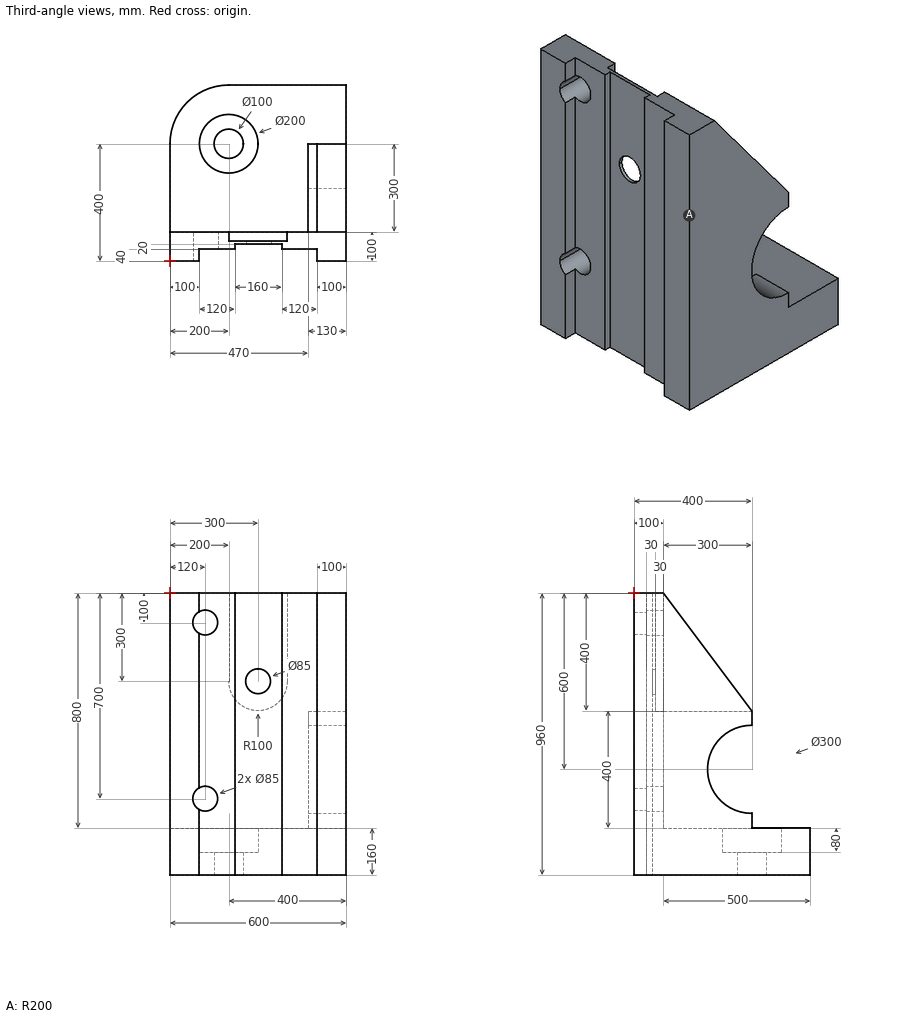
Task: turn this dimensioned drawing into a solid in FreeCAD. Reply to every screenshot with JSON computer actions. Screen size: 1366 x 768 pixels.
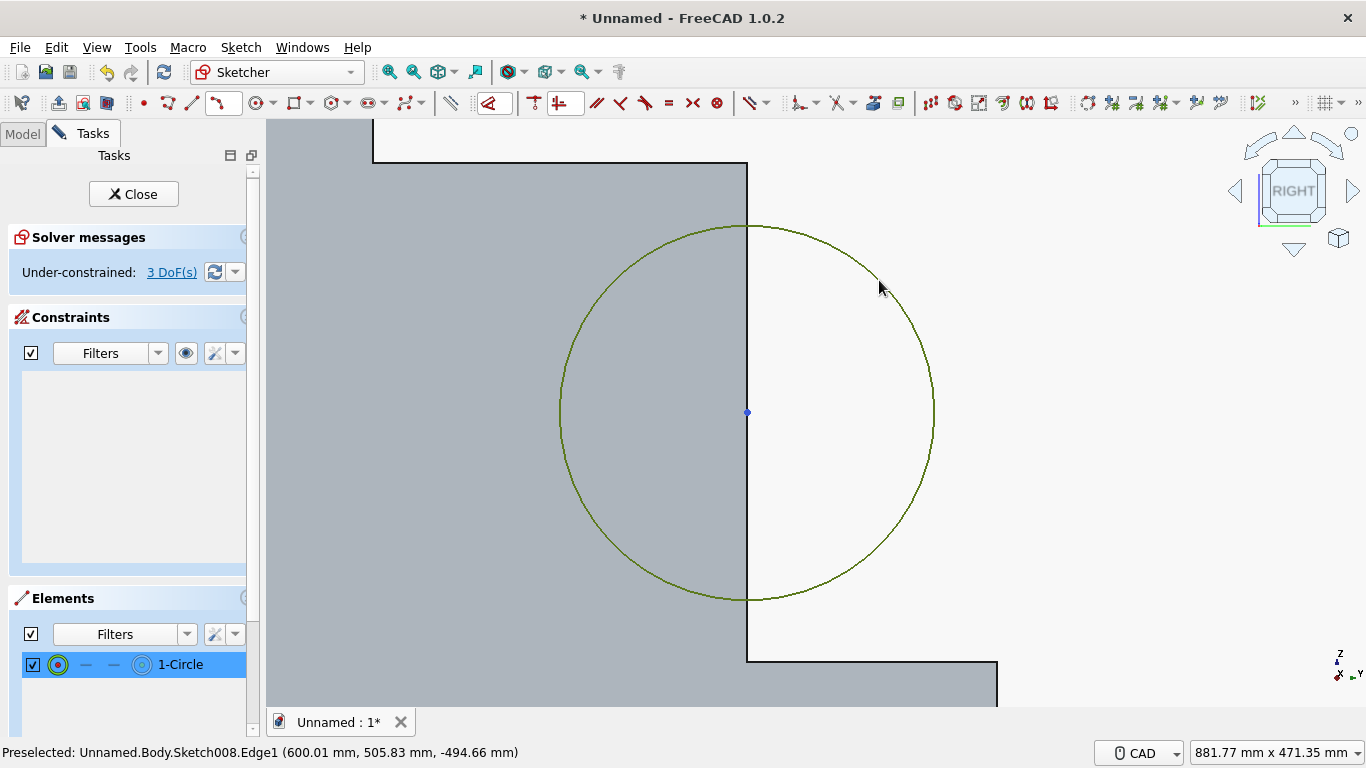
{"action": "key", "text": "k o"}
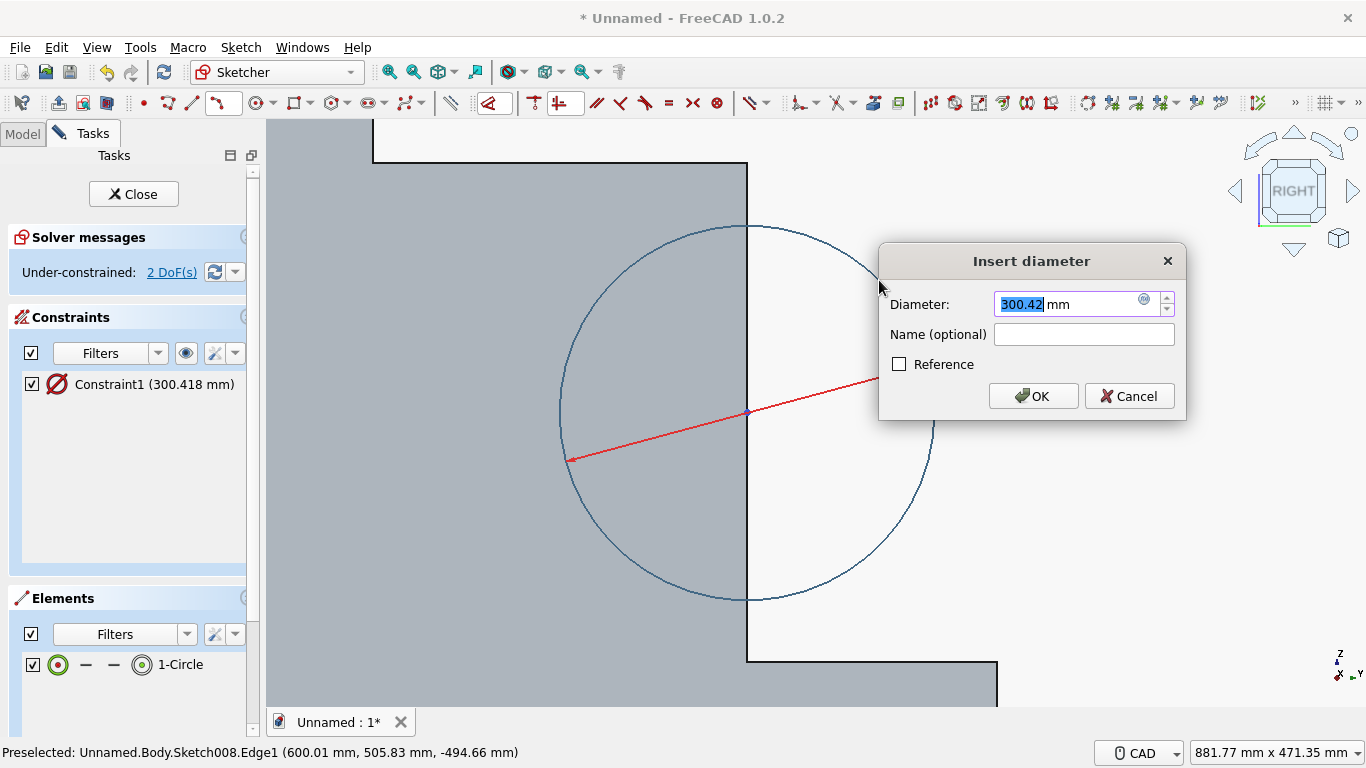
{"action": "type", "text": "300"}
{"action": "key", "text": "Return"}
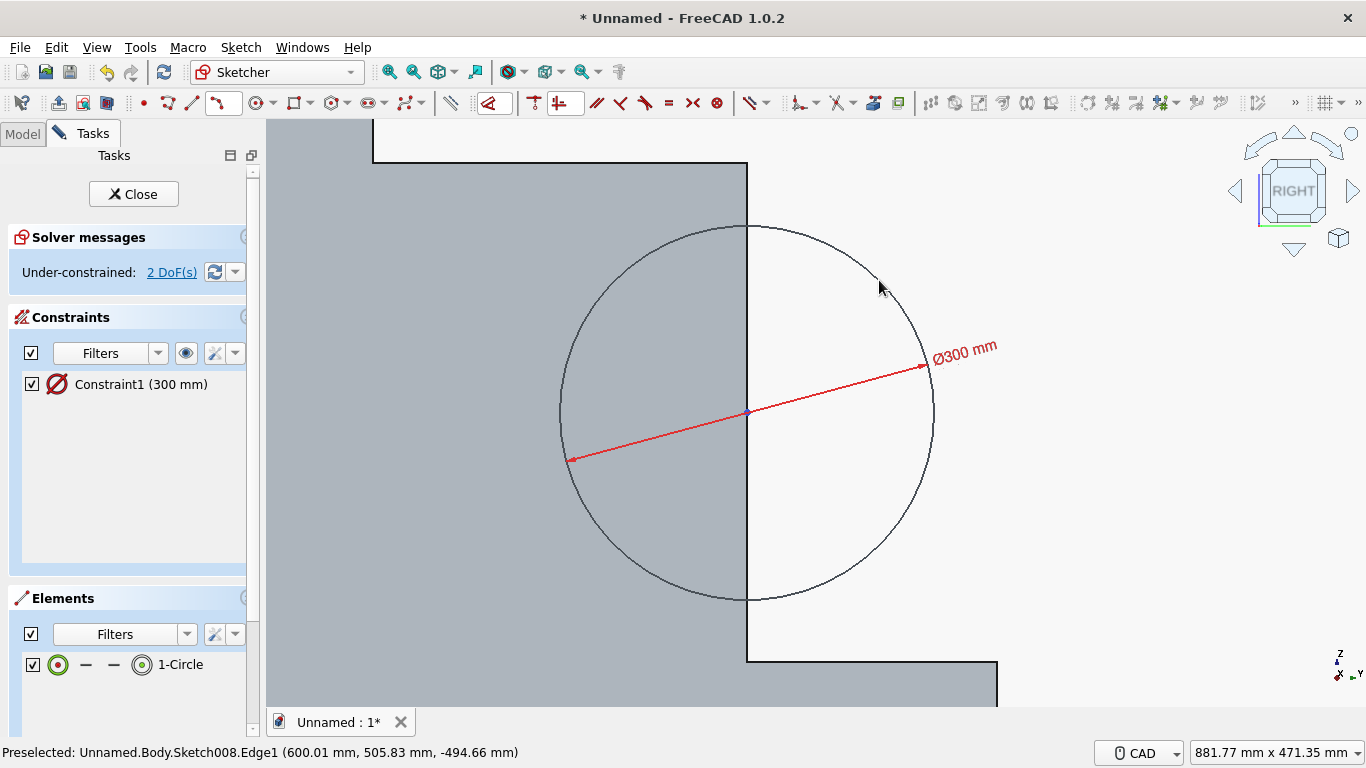
{"action": "left_click", "coordinate": [747, 413]}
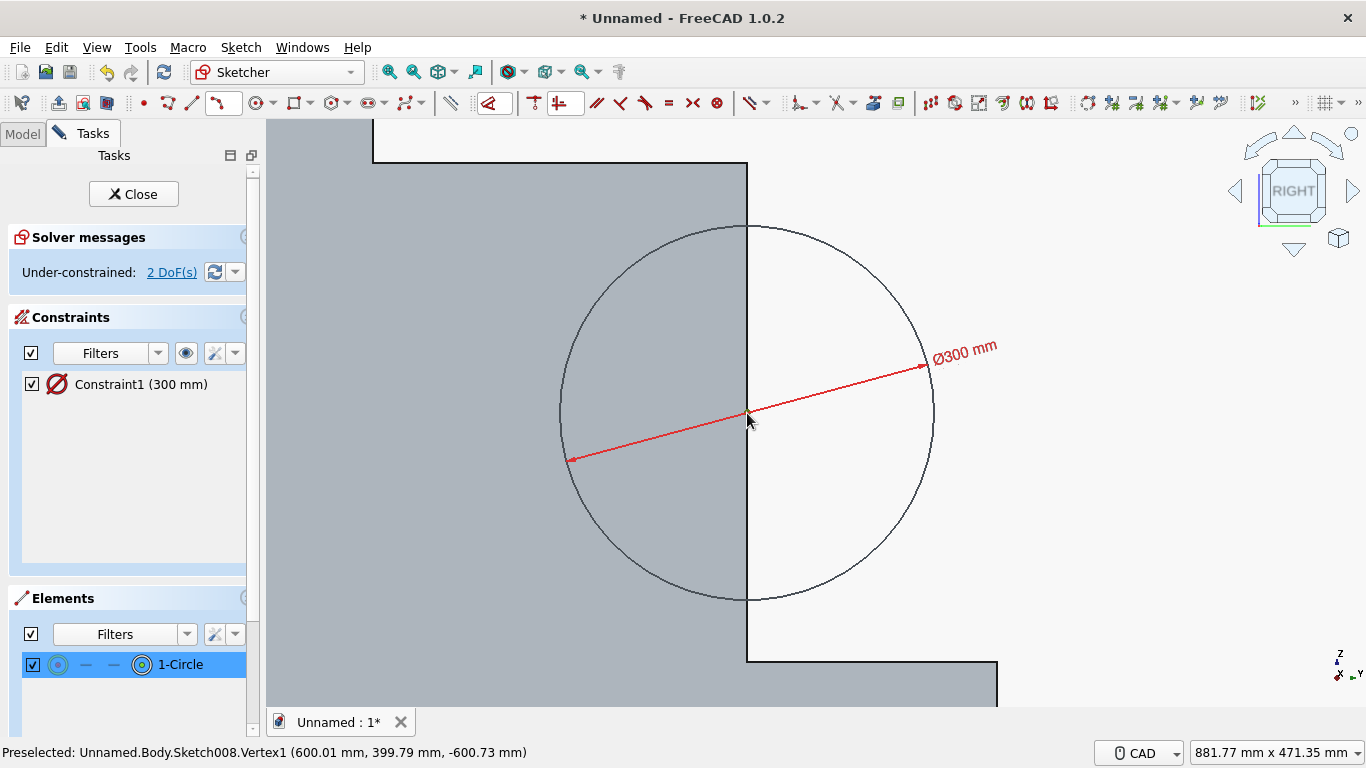
{"action": "key", "text": "l"}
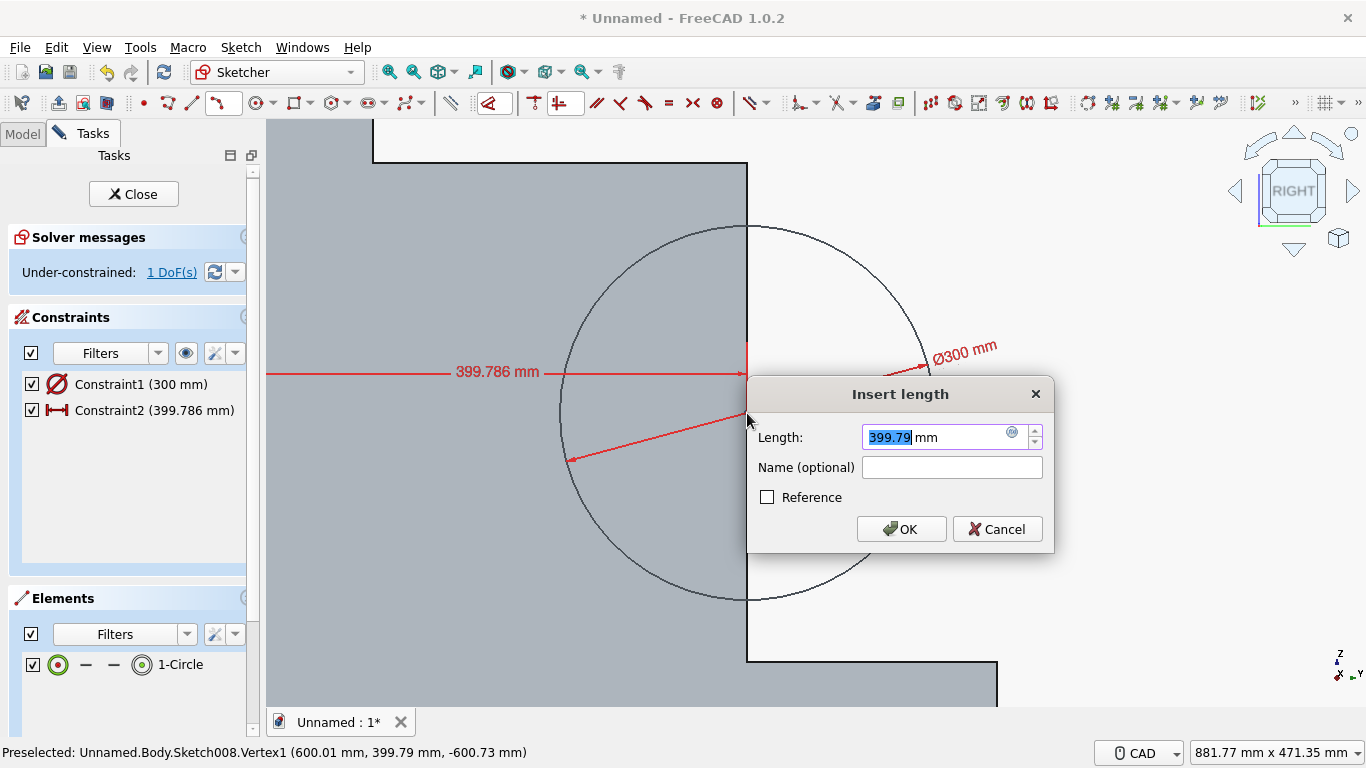
{"action": "type", "text": "400"}
{"action": "key", "text": "Return"}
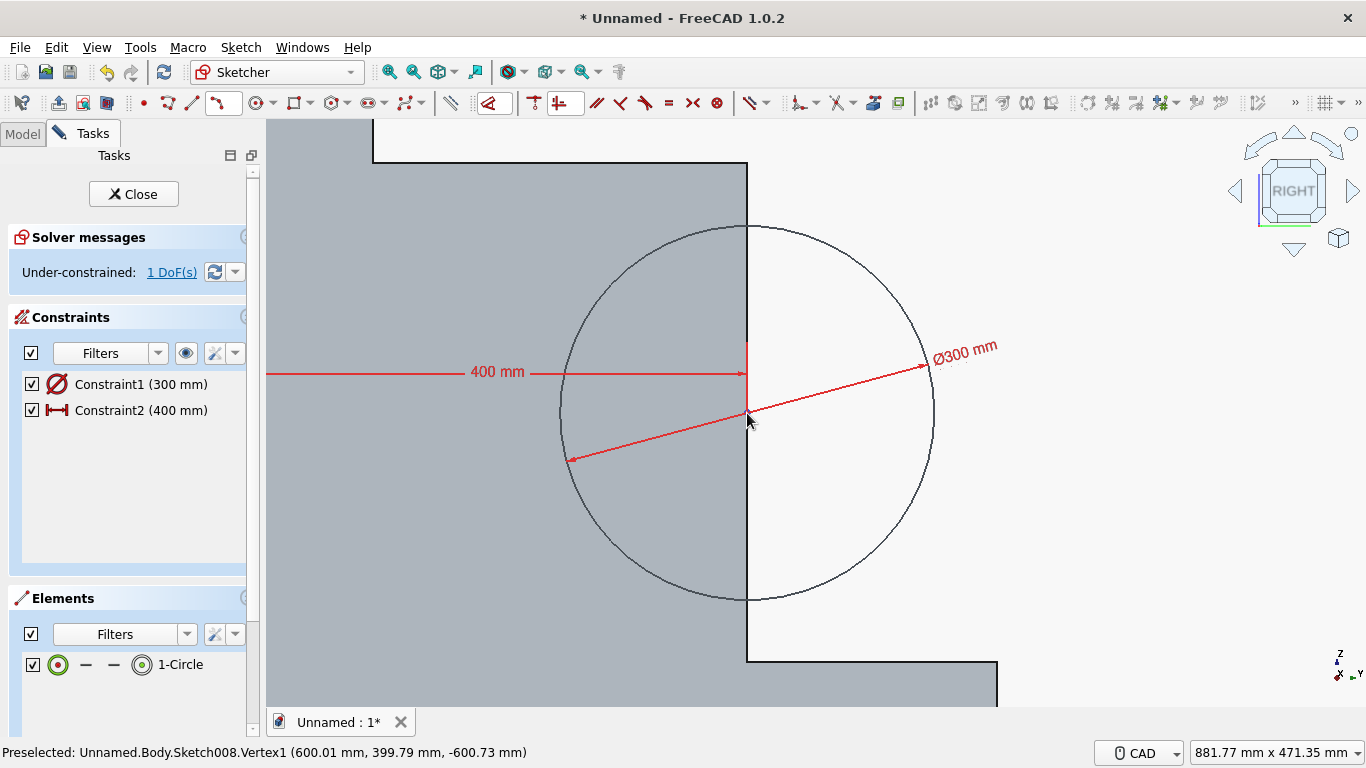
{"action": "left_click", "coordinate": [747, 413]}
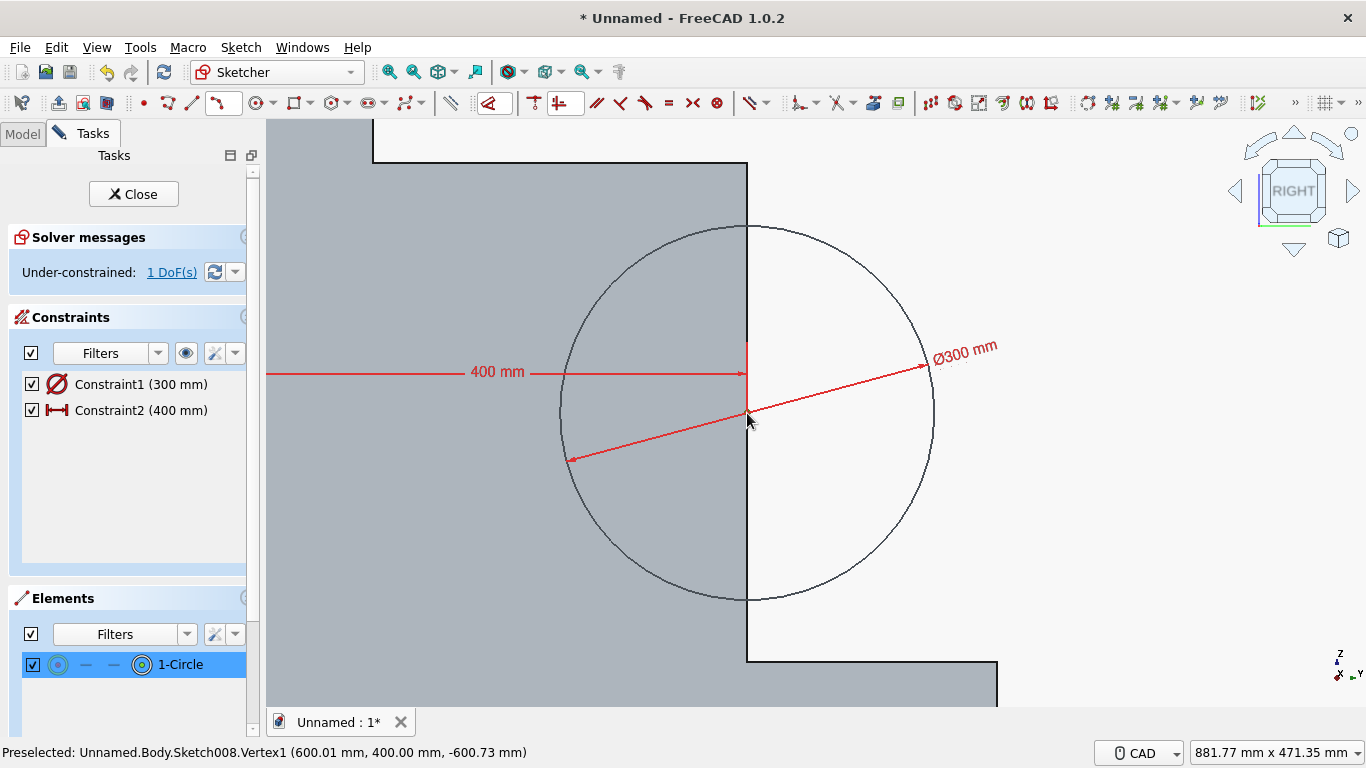
{"action": "left_click", "coordinate": [506, 104]}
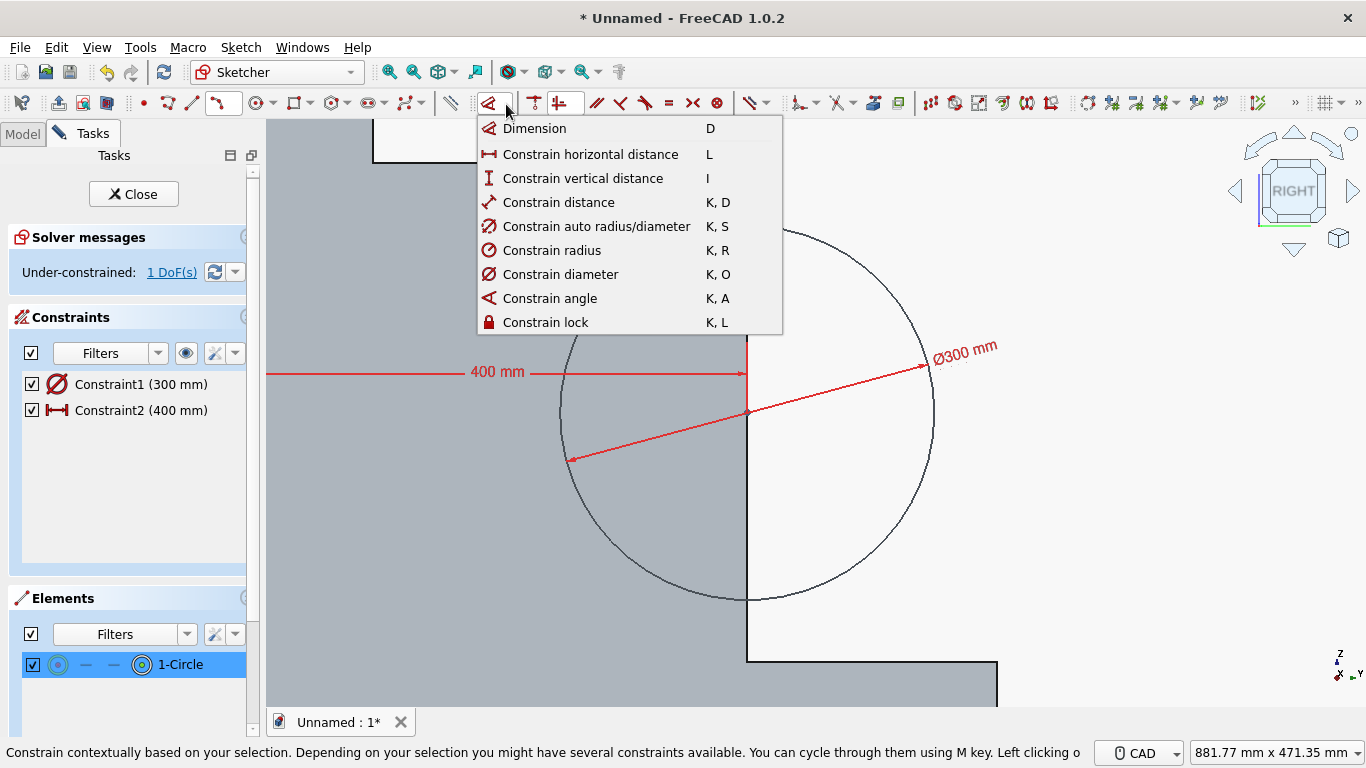
{"action": "left_click", "coordinate": [630, 178]}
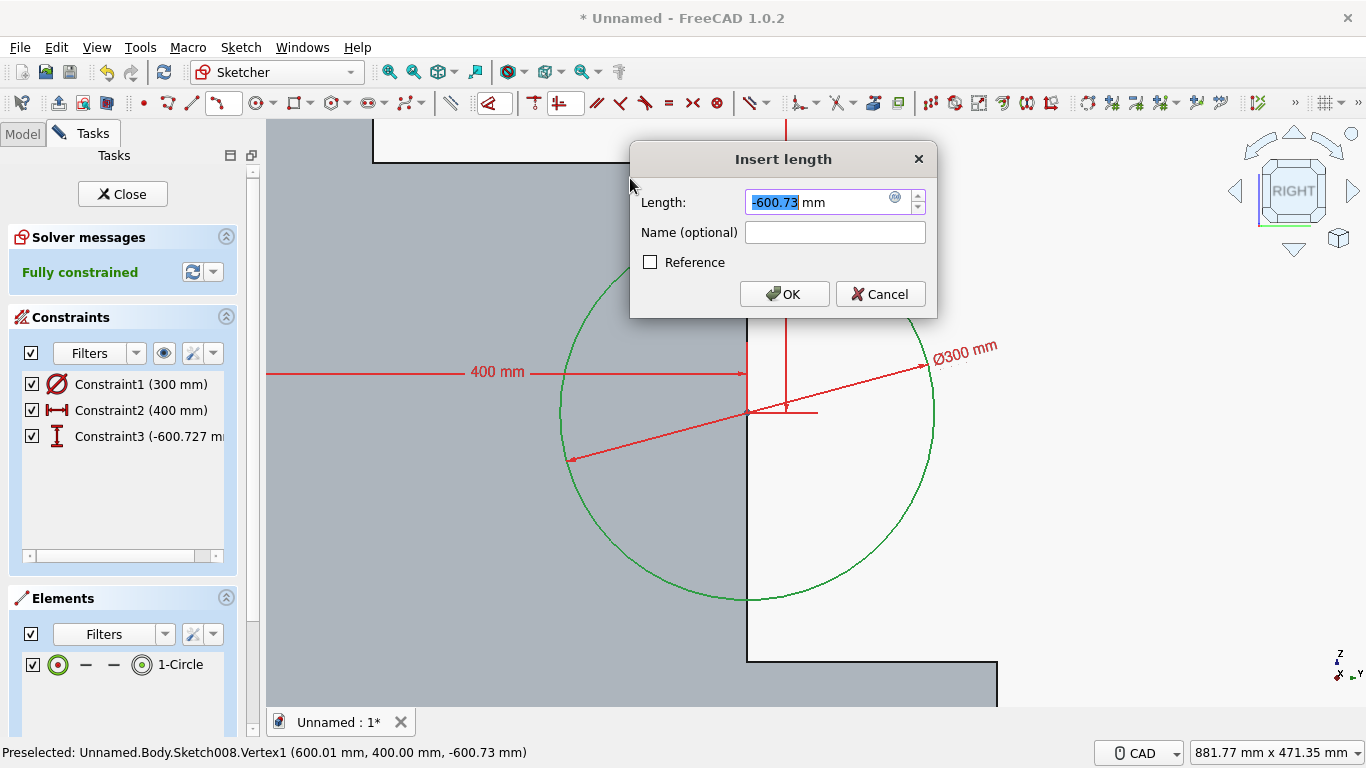
{"action": "type", "text": "-600"}
{"action": "key", "text": "Return"}